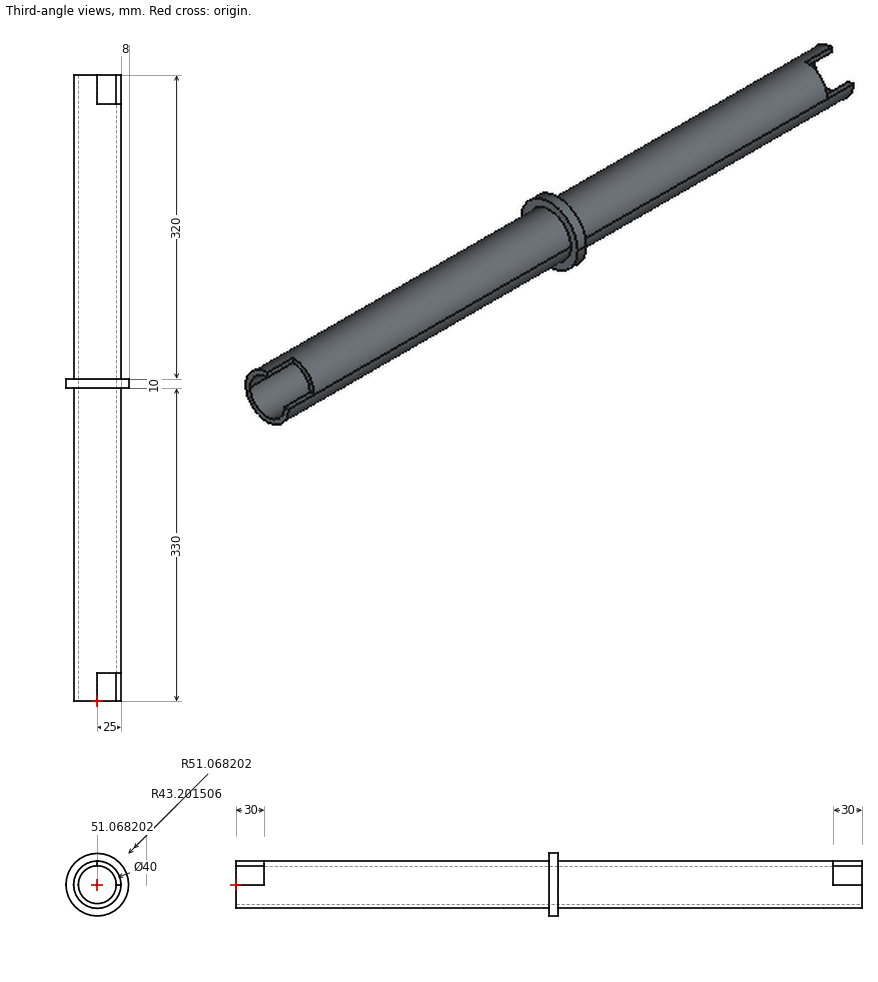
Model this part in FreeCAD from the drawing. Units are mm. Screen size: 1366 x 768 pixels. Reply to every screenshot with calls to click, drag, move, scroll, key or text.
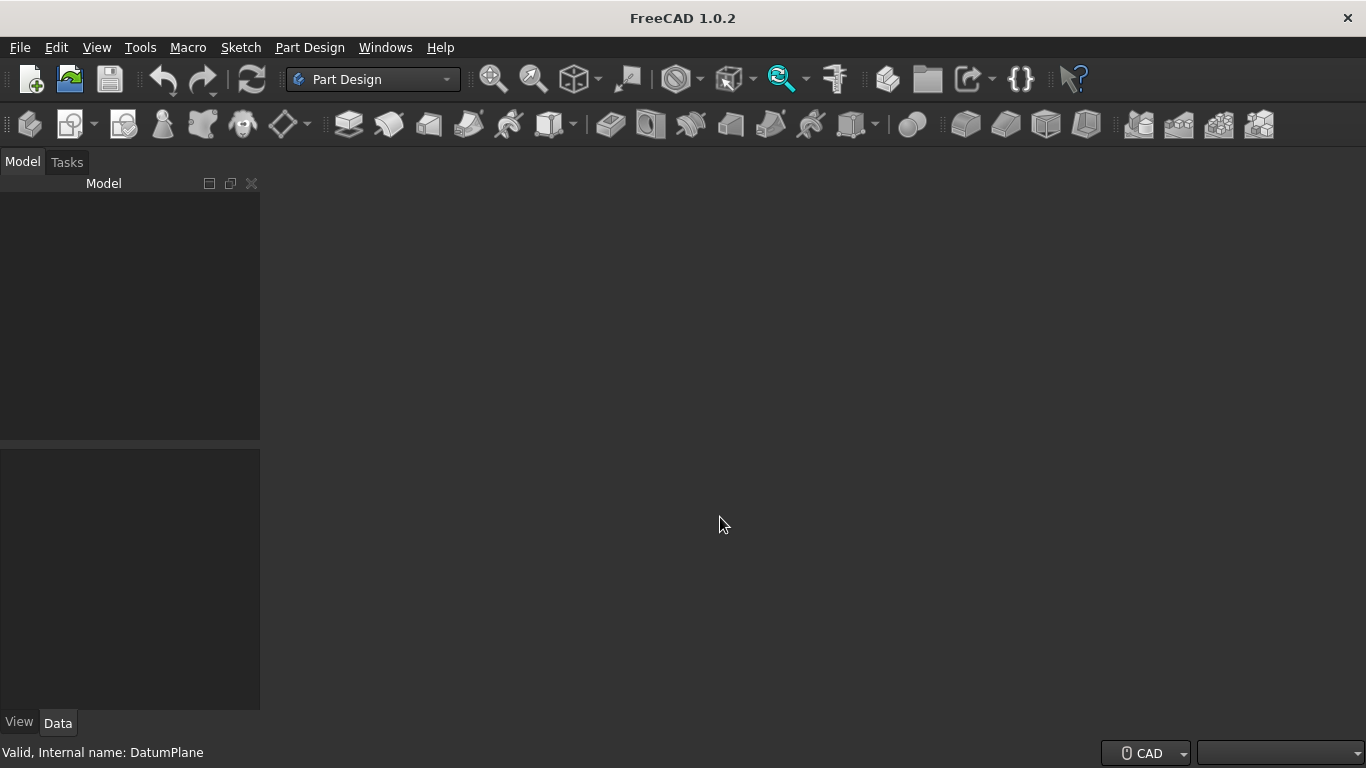
click(30, 80)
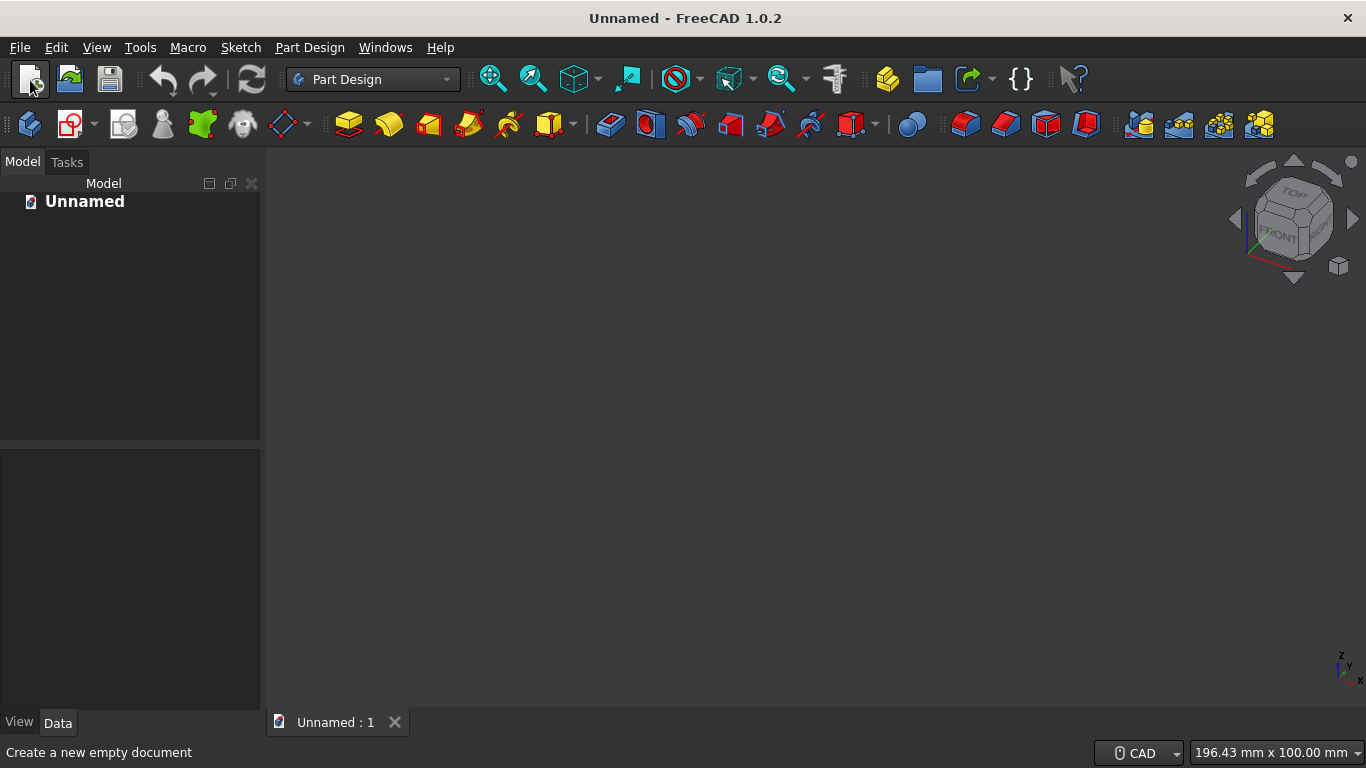
click(70, 124)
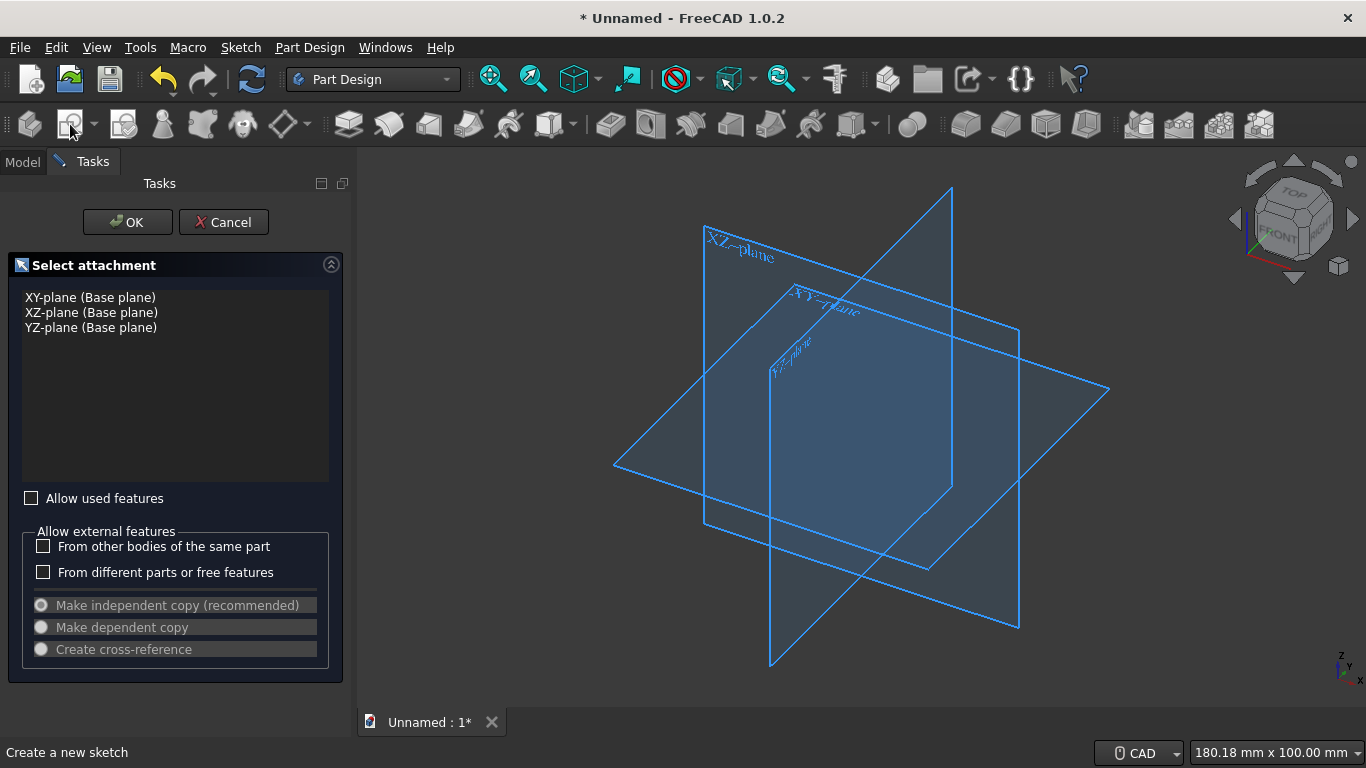
click(82, 298)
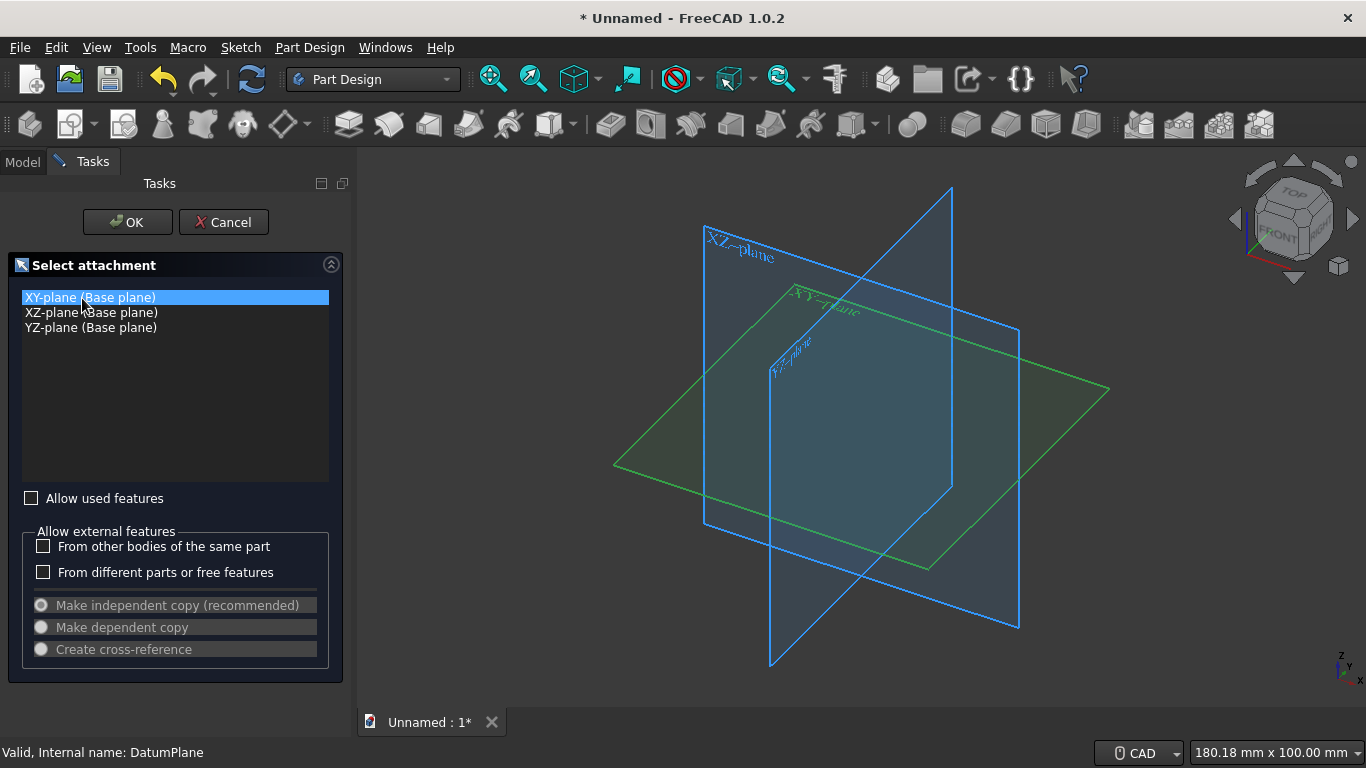
click(128, 222)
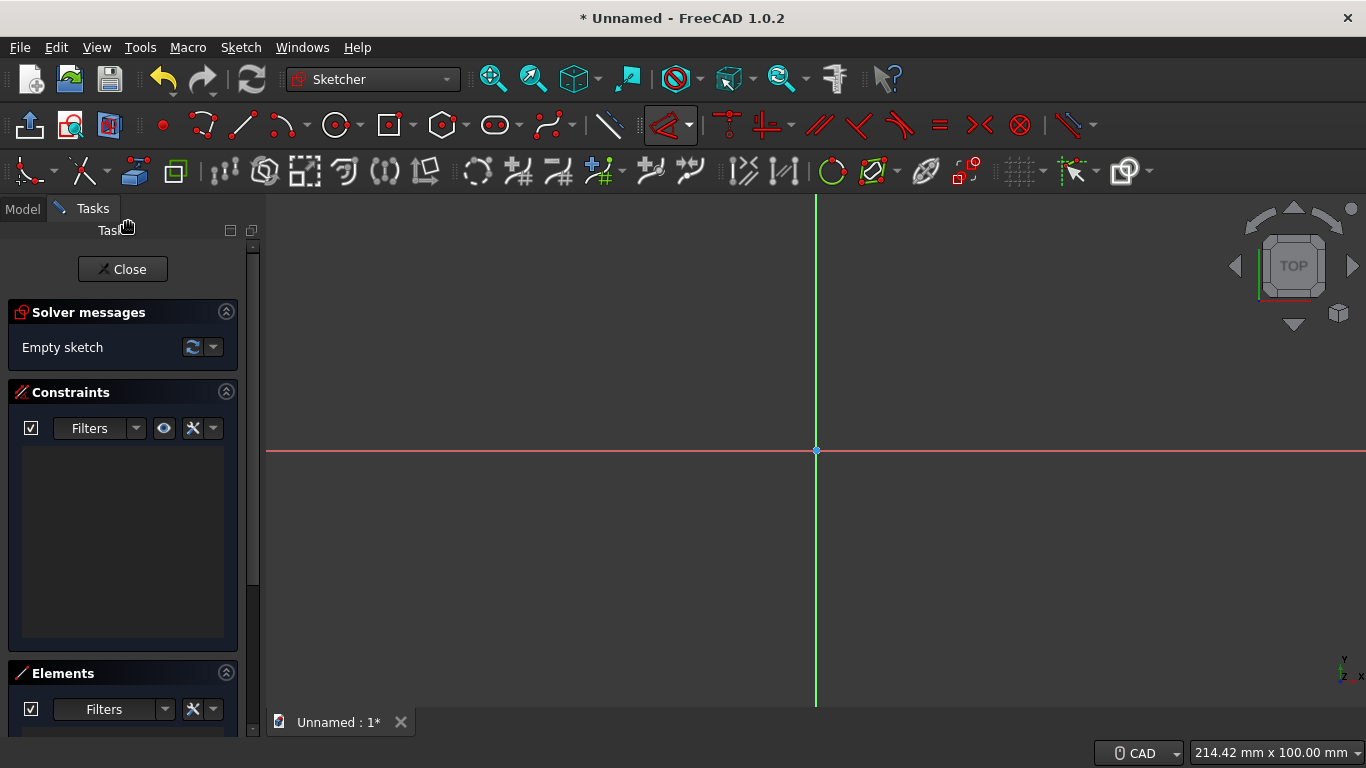
scroll(732, 619, down, 12)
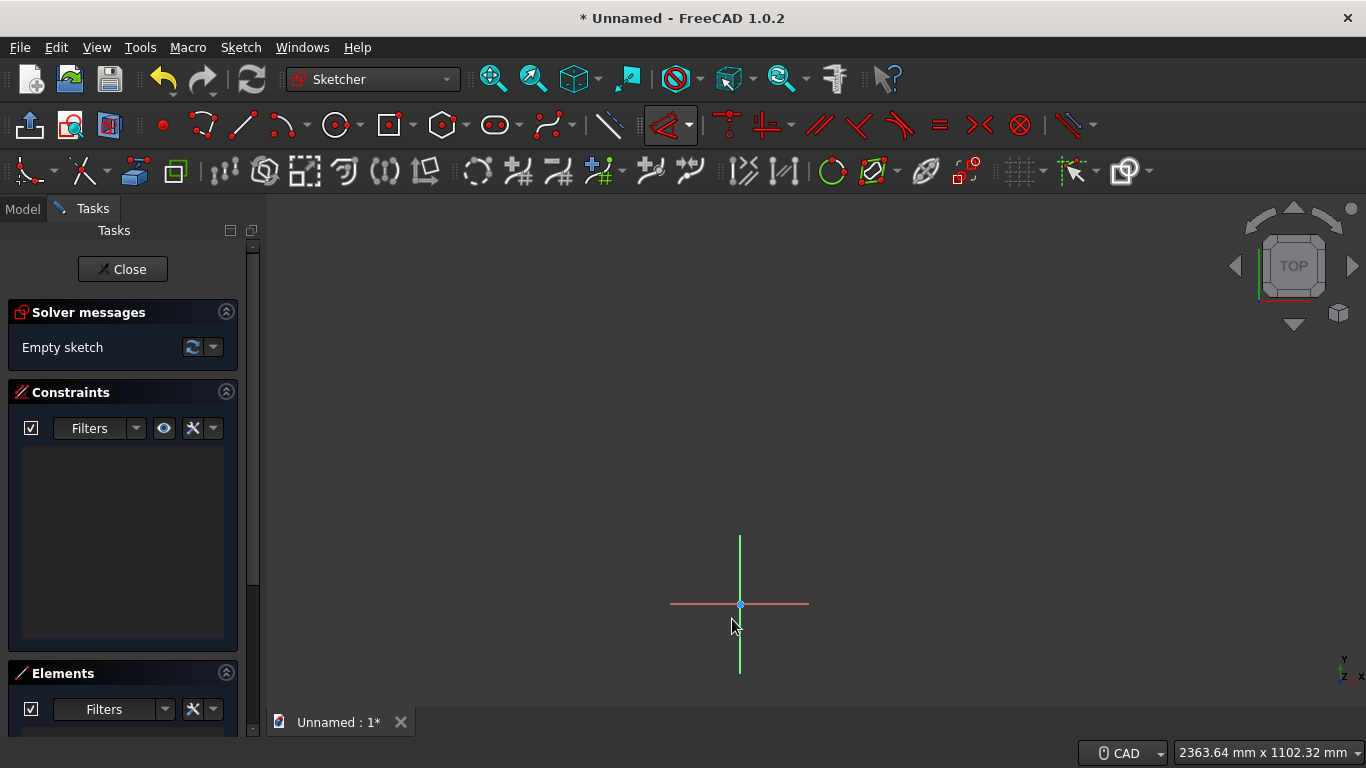
click(204, 126)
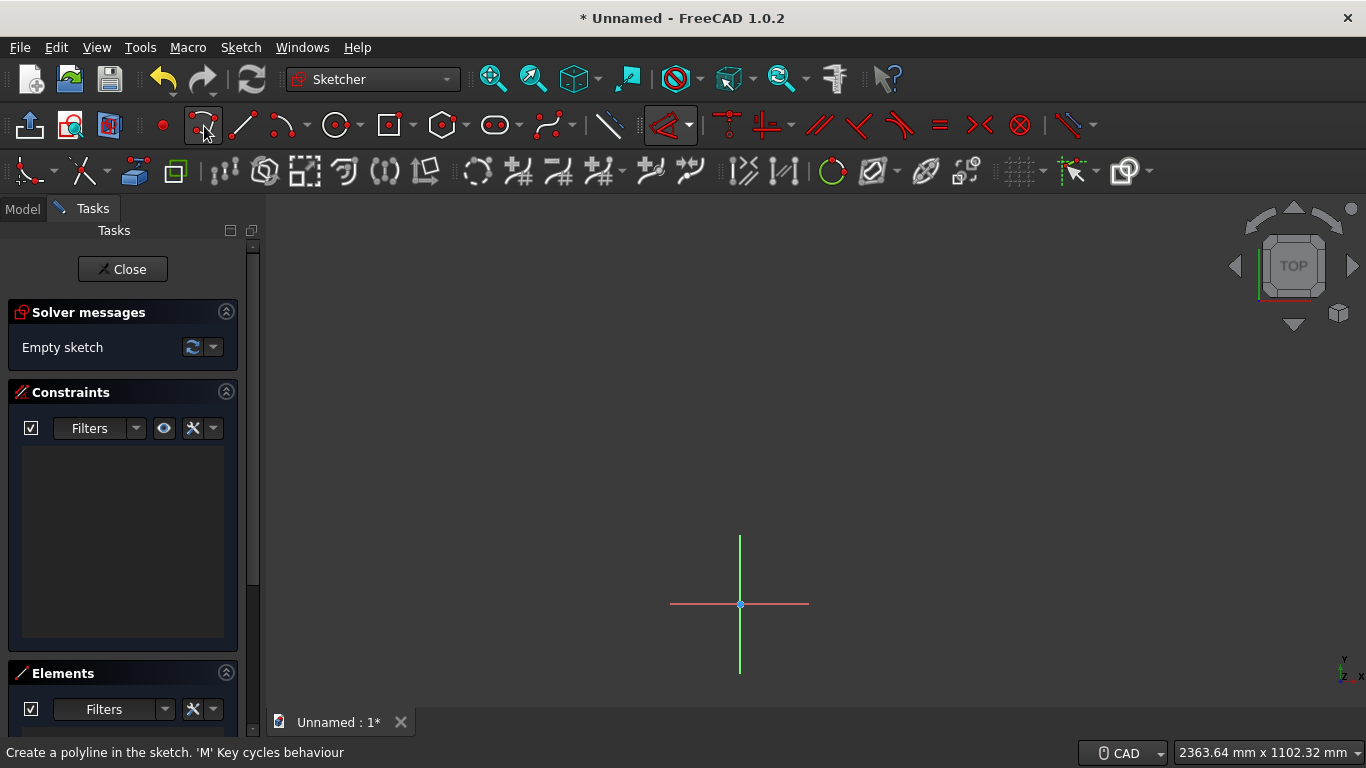
click(740, 604)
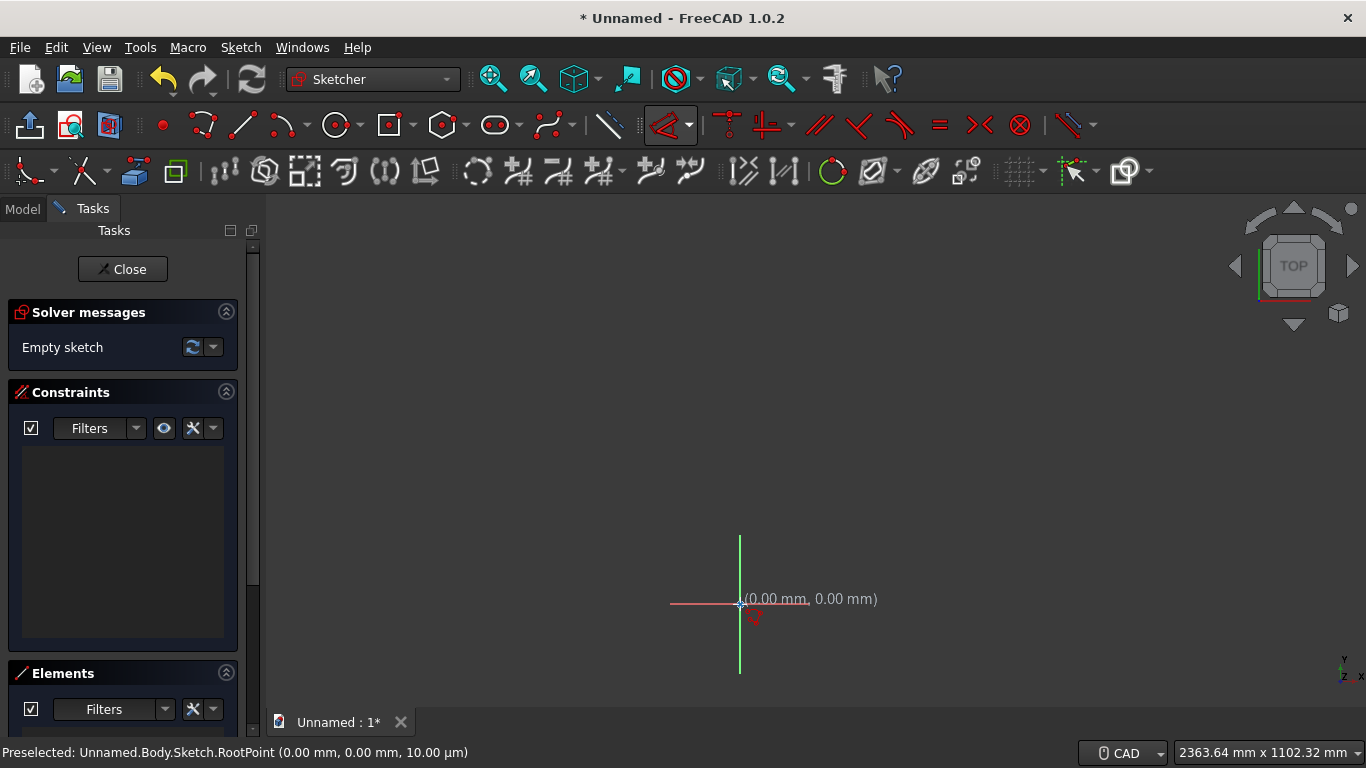
scroll(752, 604, up, 2)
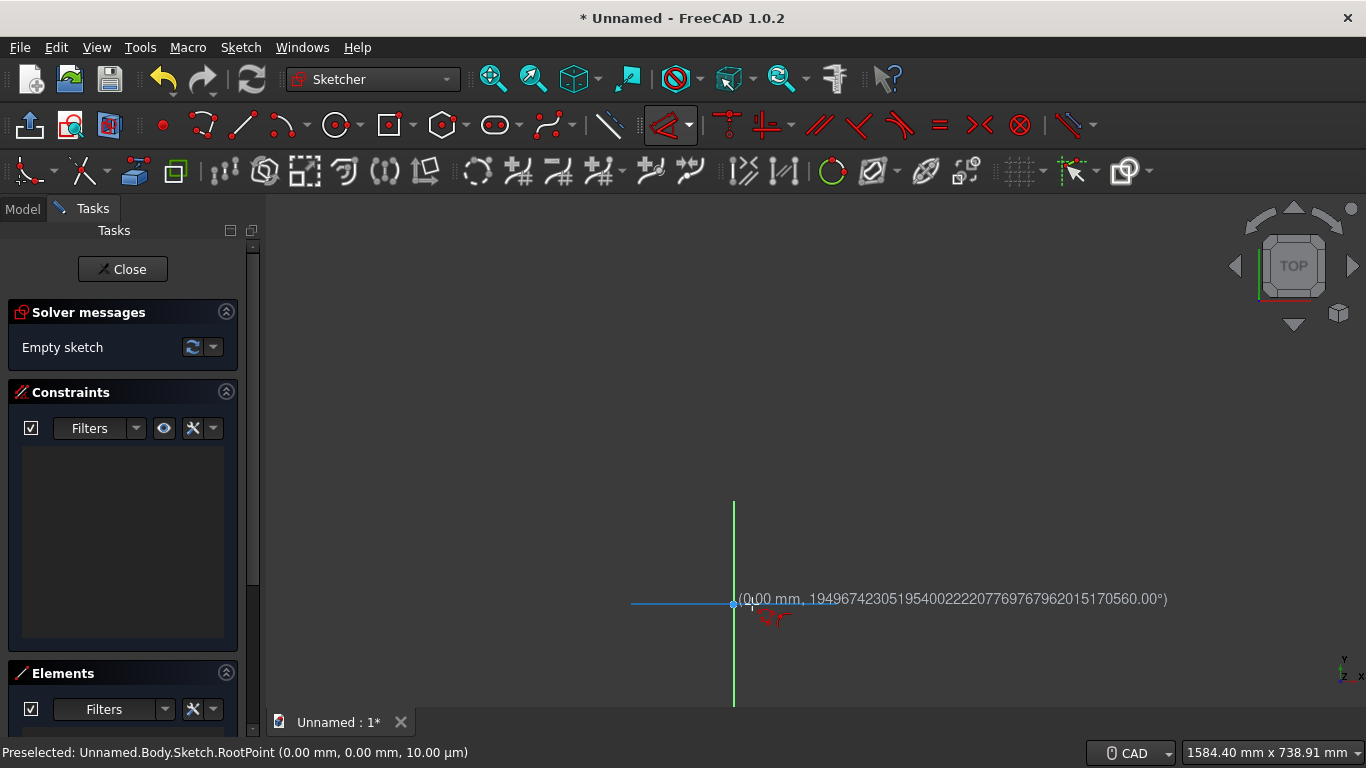
click(751, 595)
click(751, 375)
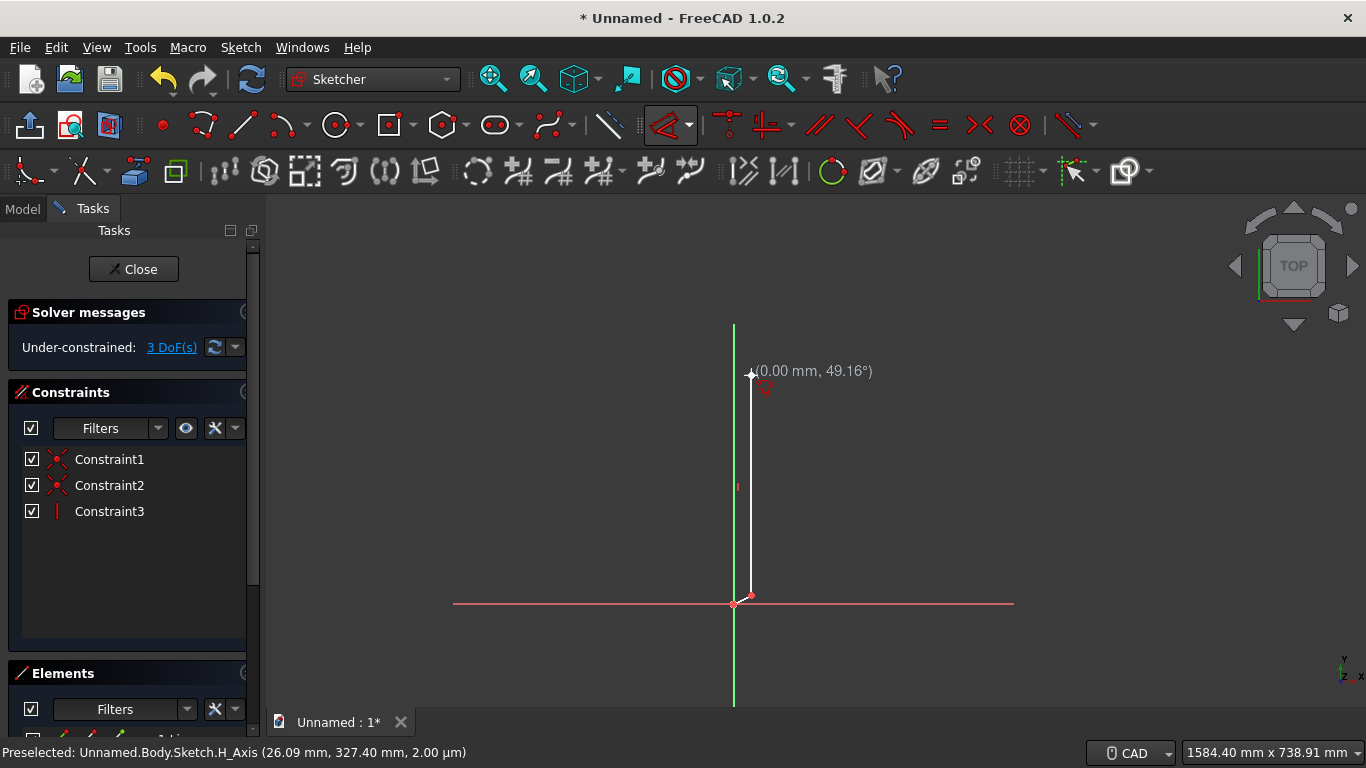
scroll(757, 375, up, 6)